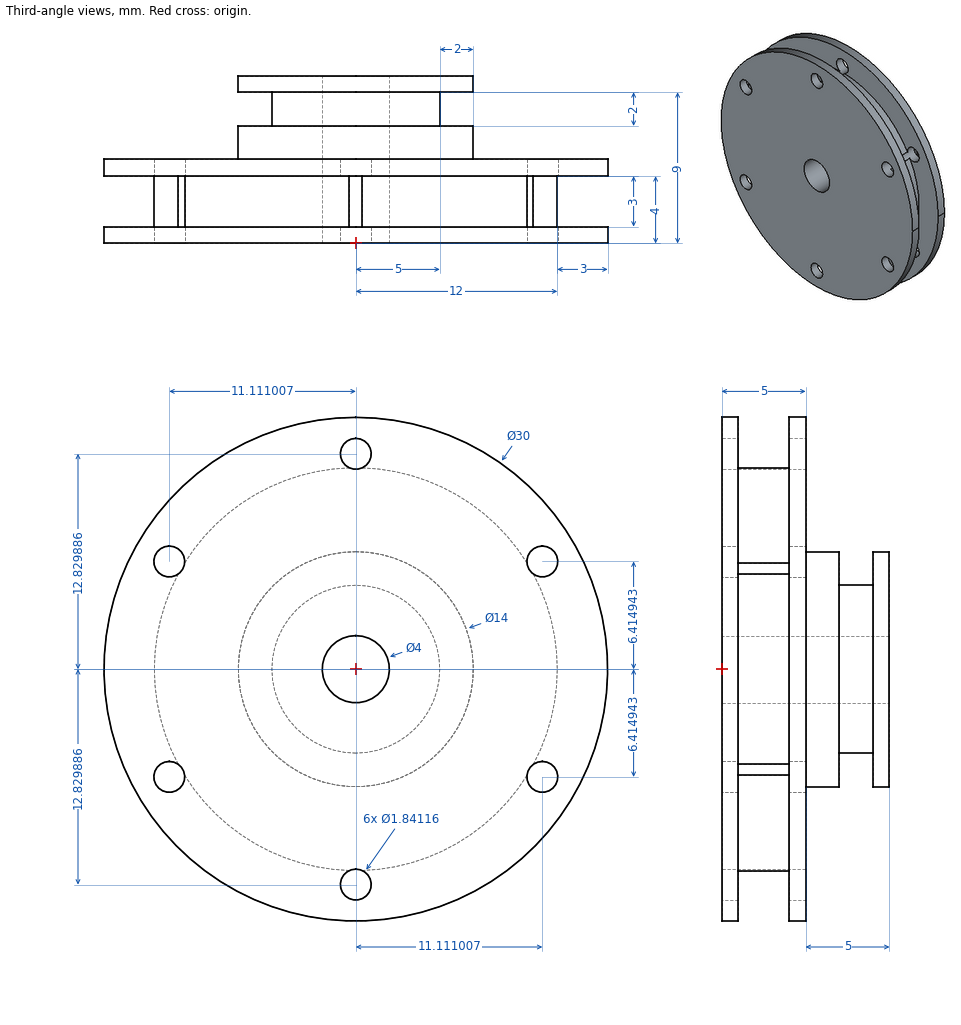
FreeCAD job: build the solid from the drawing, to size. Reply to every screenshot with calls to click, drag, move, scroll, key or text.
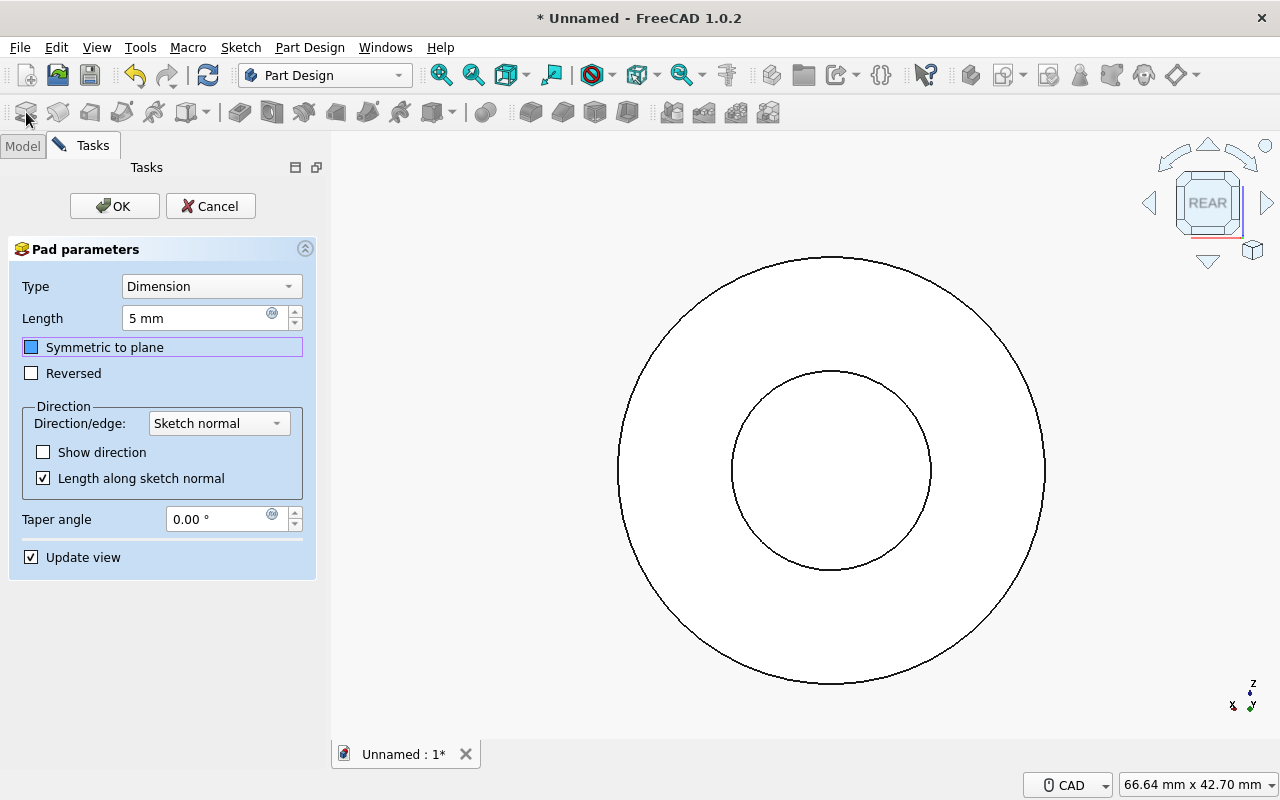
click(115, 206)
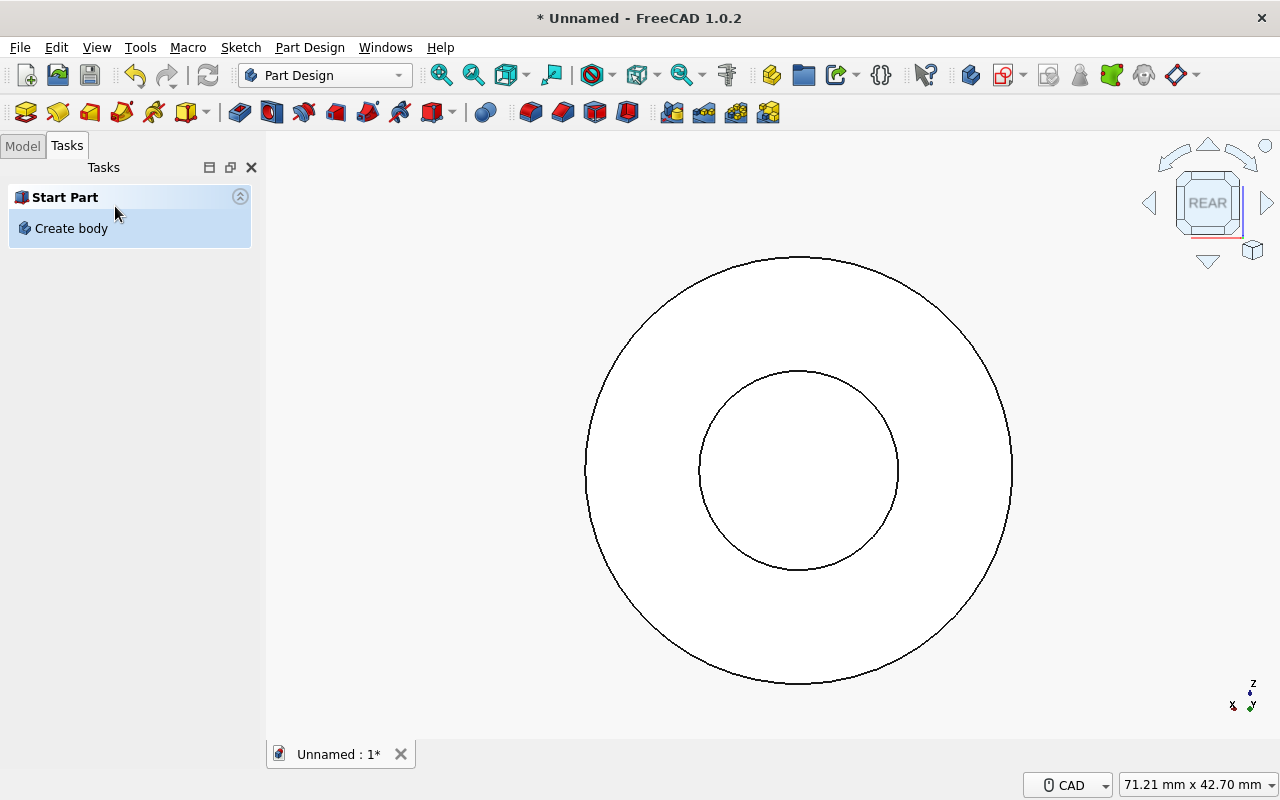
click(1004, 76)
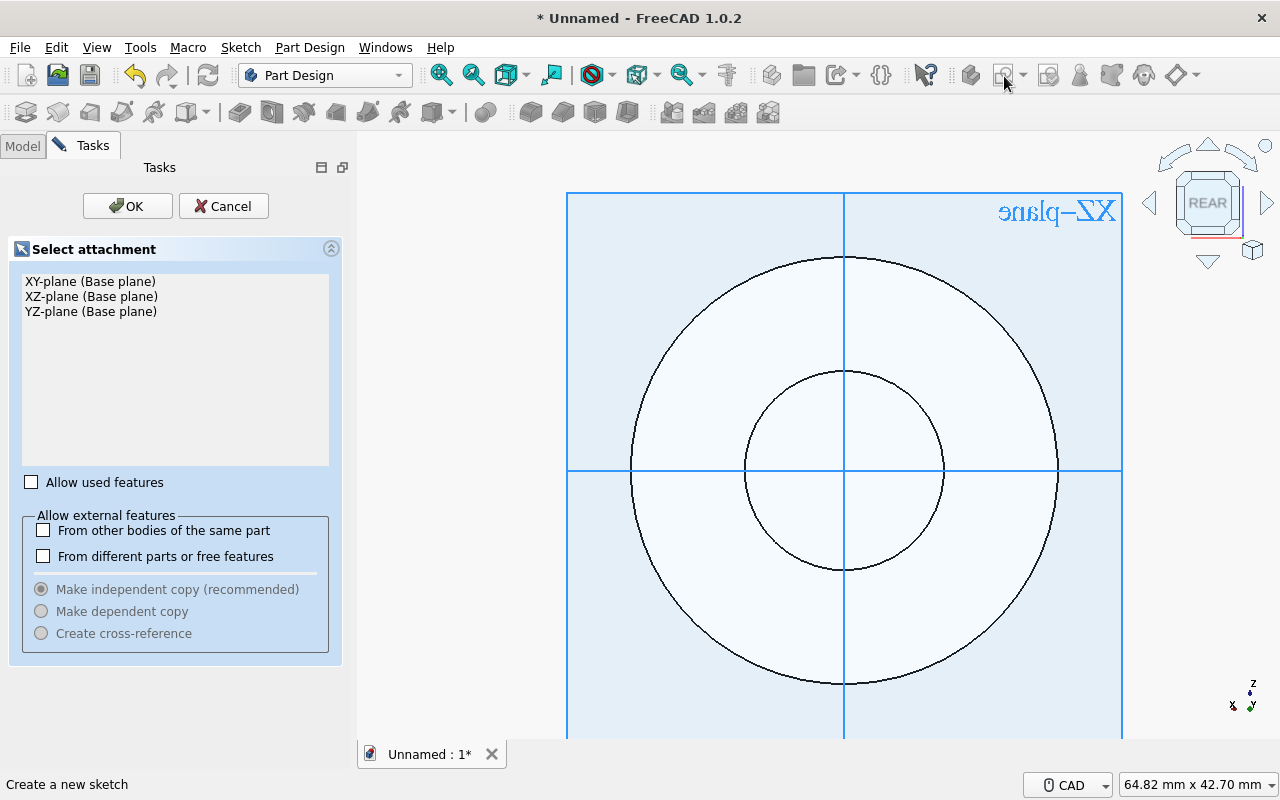
click(82, 282)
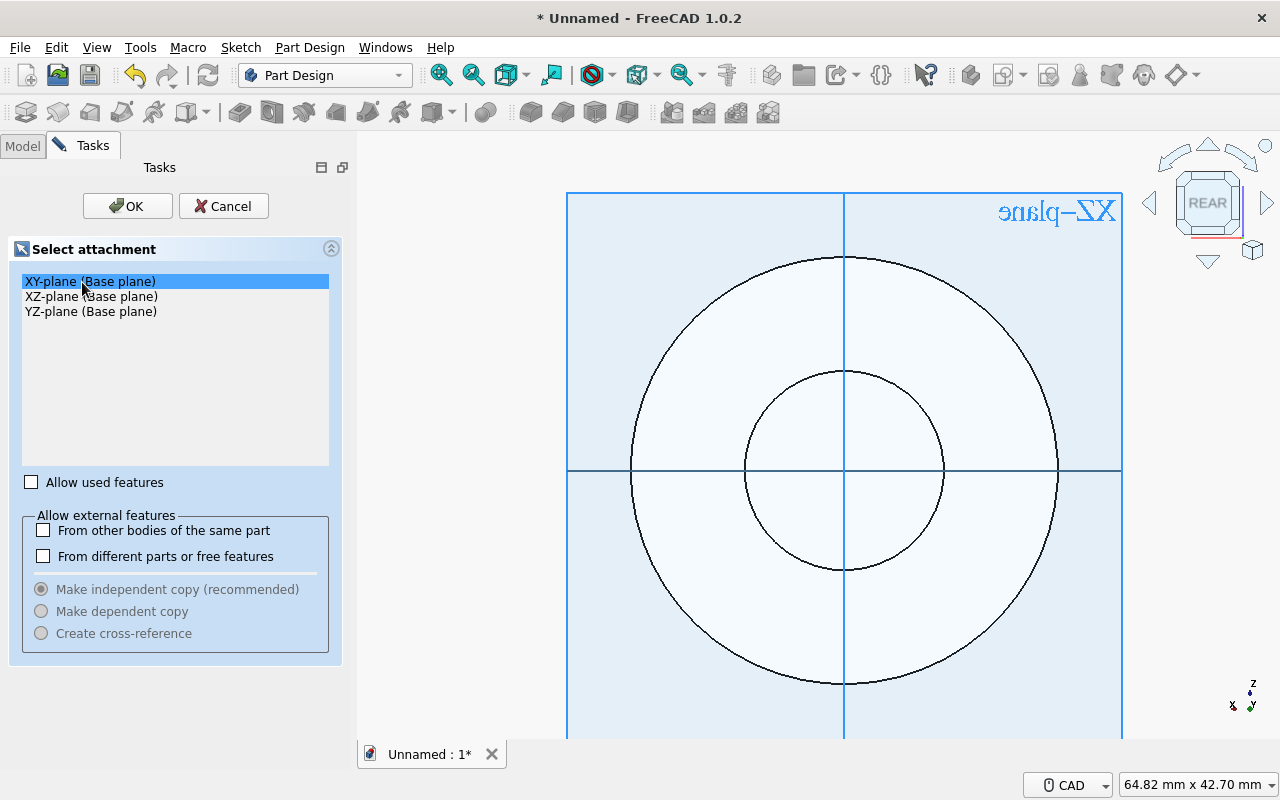
click(128, 206)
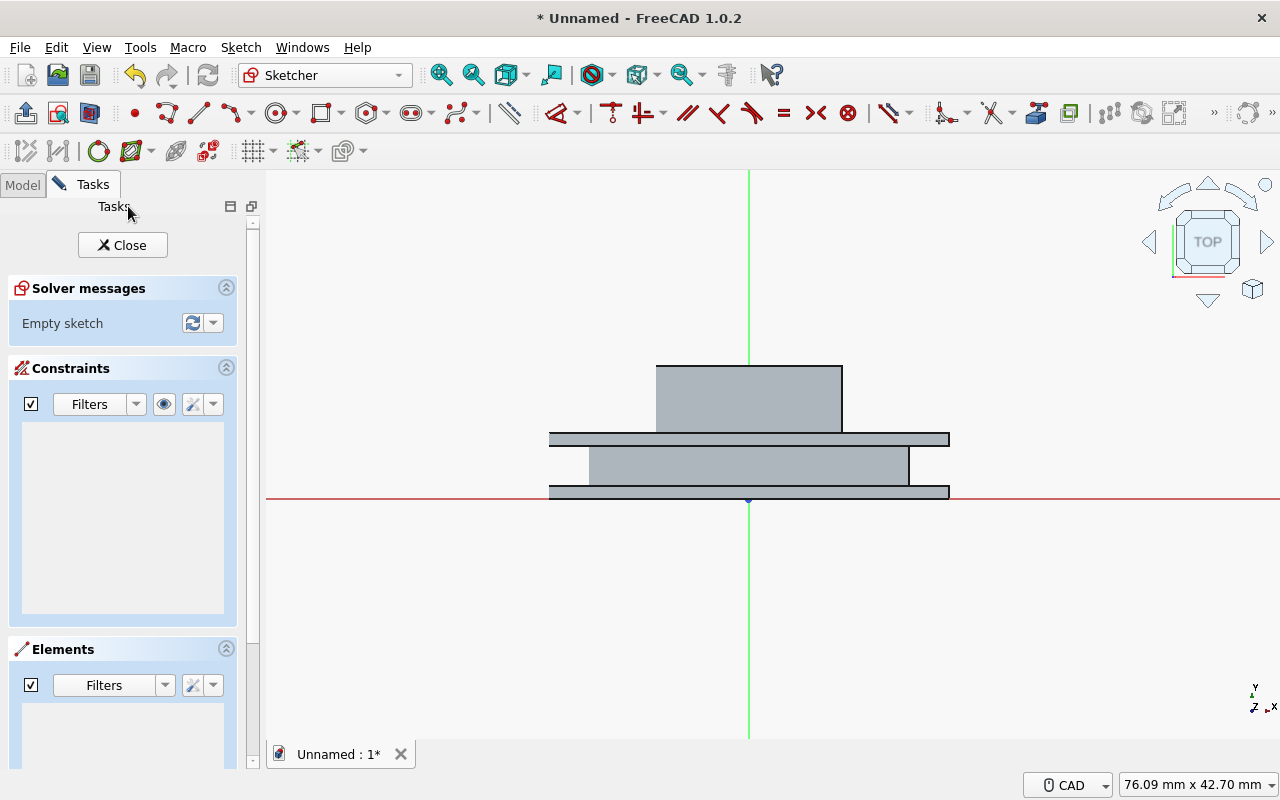
click(90, 114)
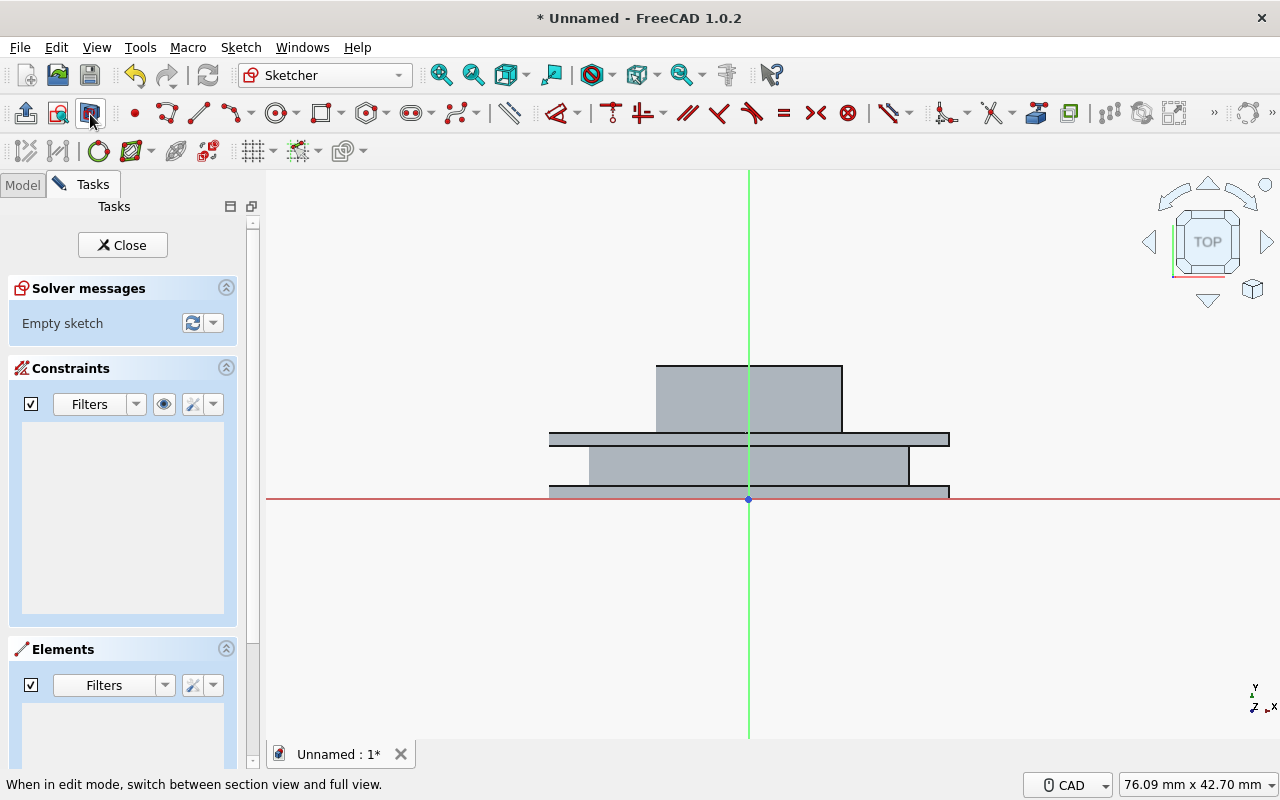
scroll(839, 388, up, 13)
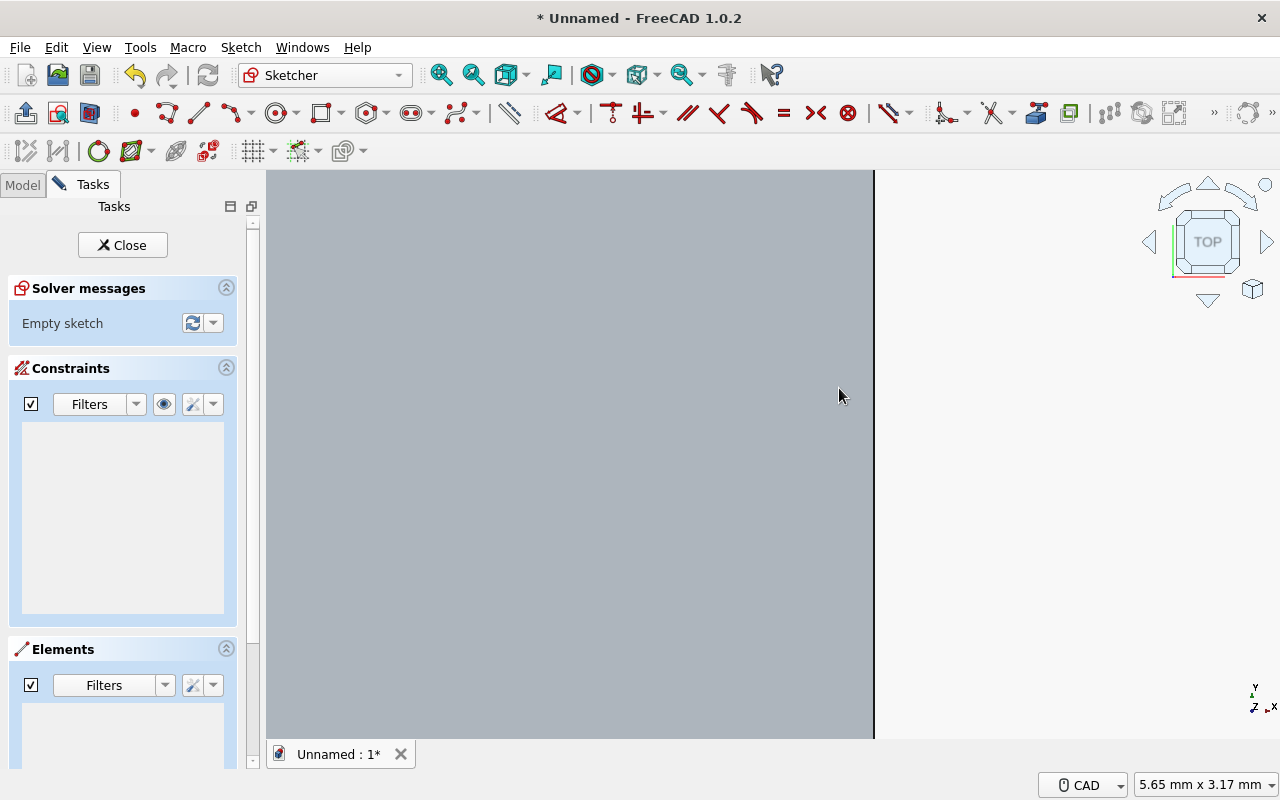
click(322, 114)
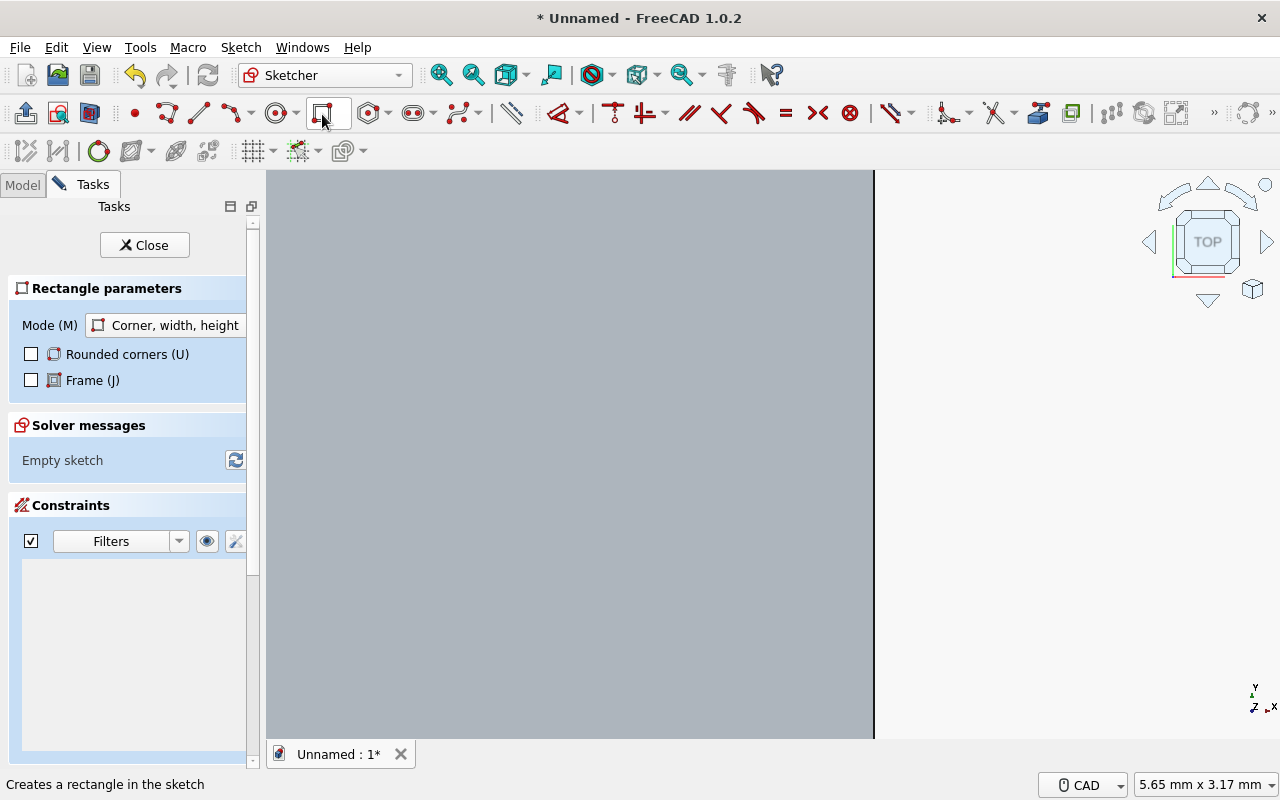
click(516, 265)
move(874, 624)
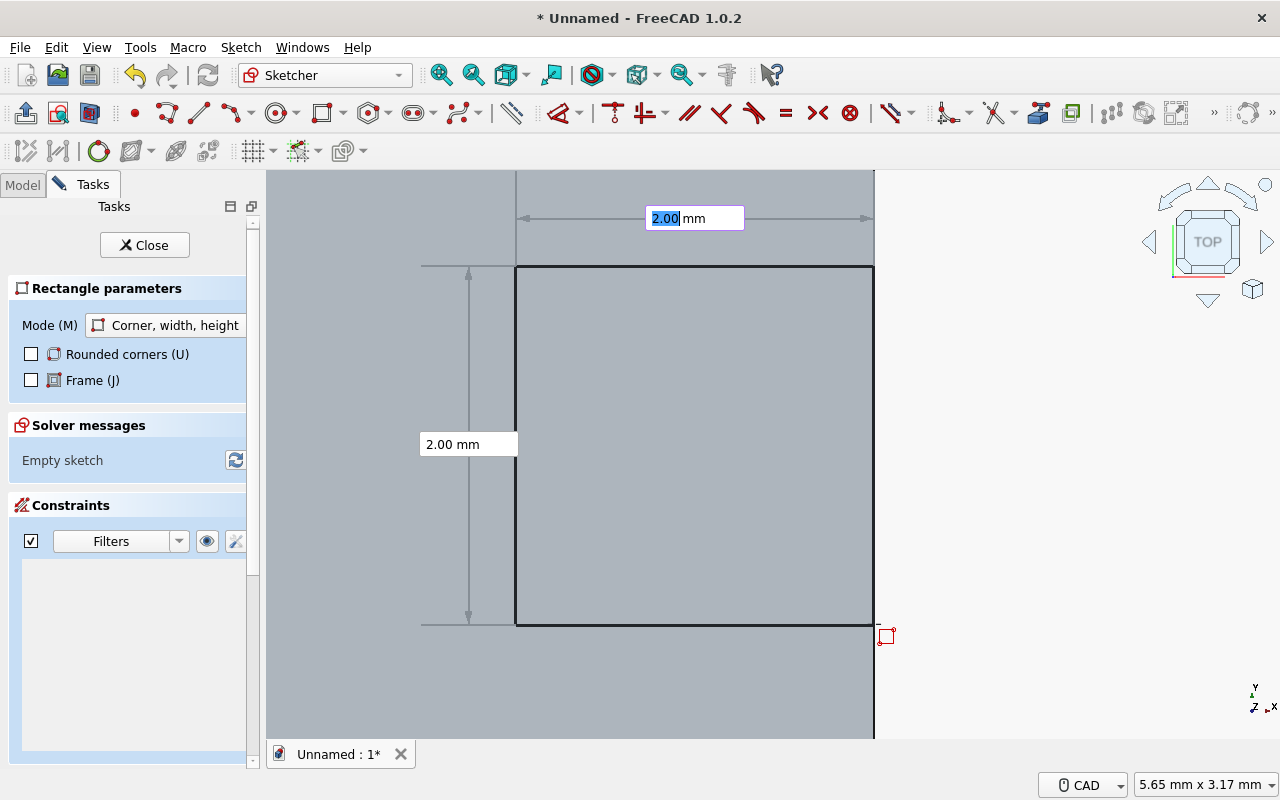
text(2)
key(Tab)
text(2)
key(Return)
key(Escape)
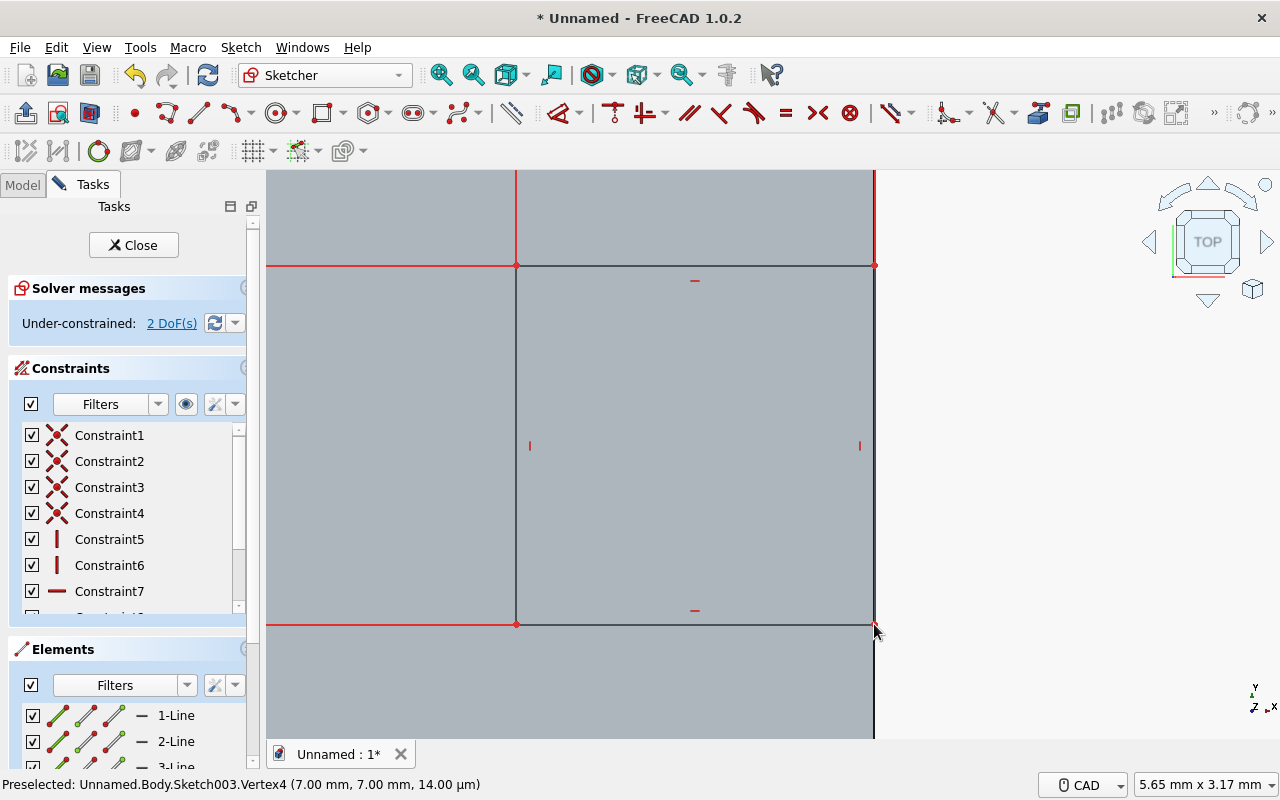
click(558, 114)